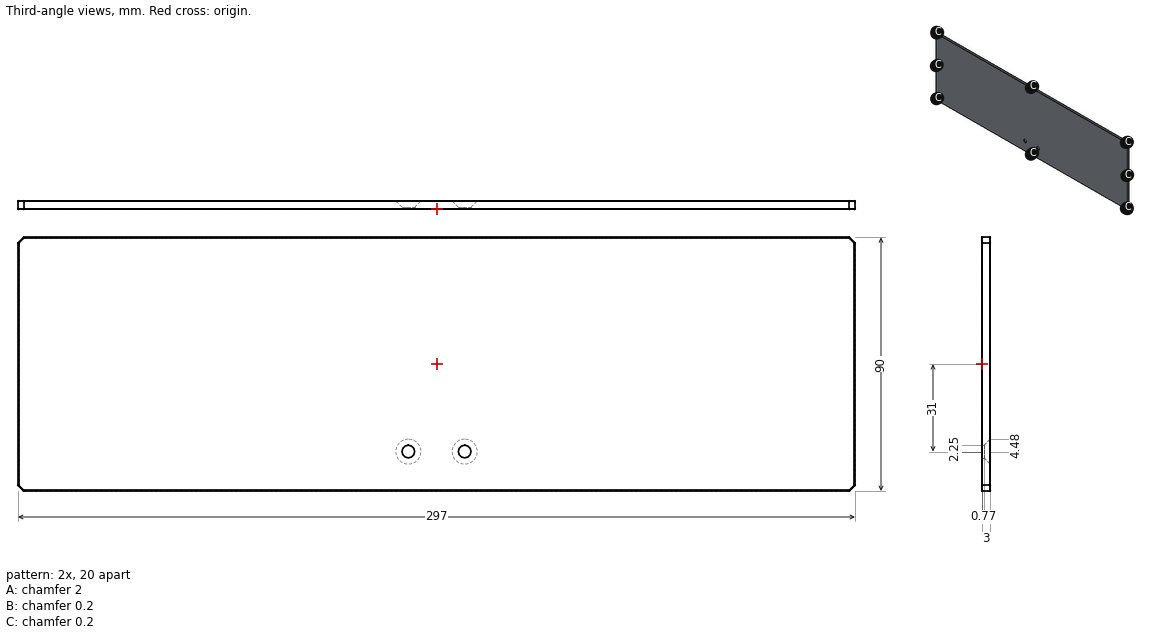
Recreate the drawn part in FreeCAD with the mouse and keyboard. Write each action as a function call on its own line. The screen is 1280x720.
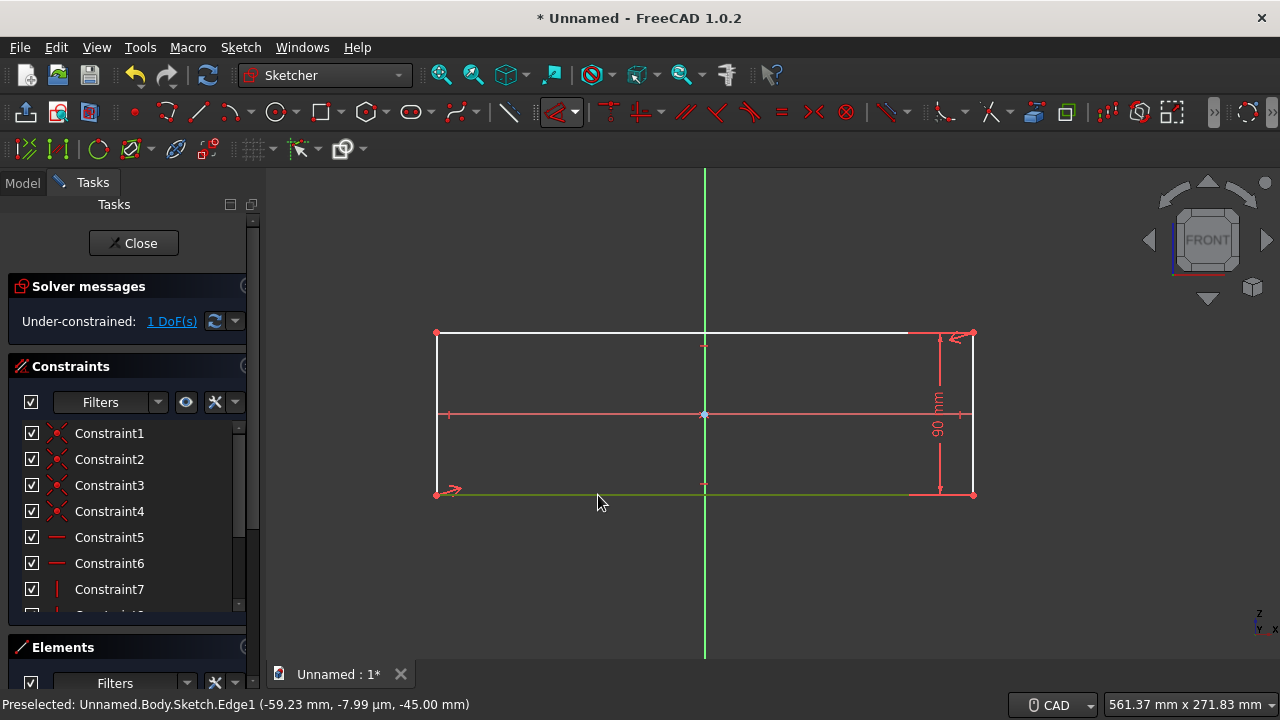
key(l)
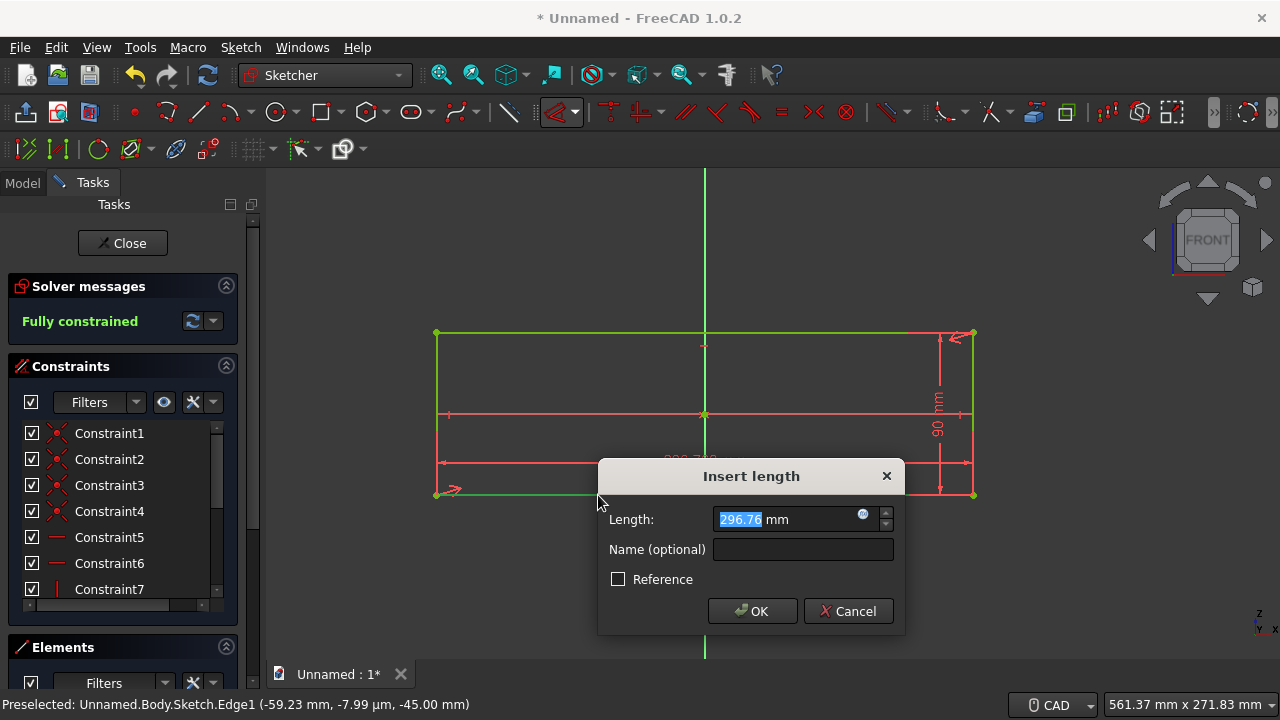
text(297)
key(Return)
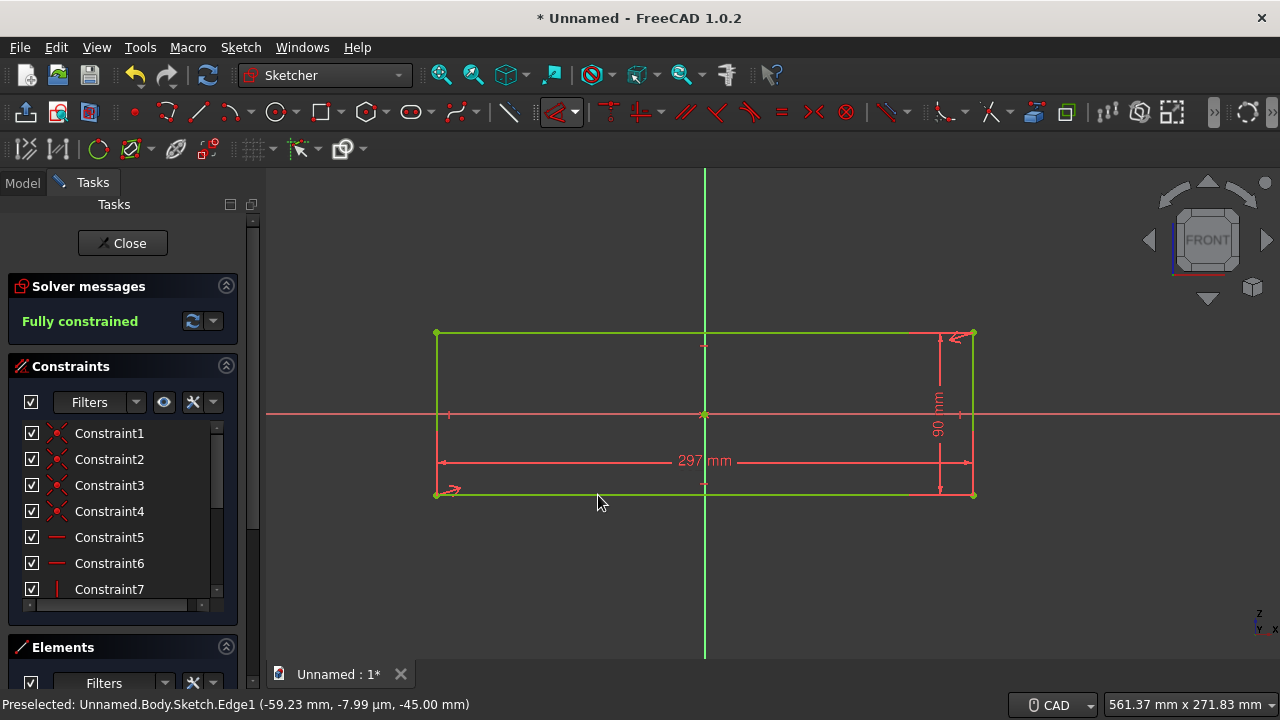
click(123, 243)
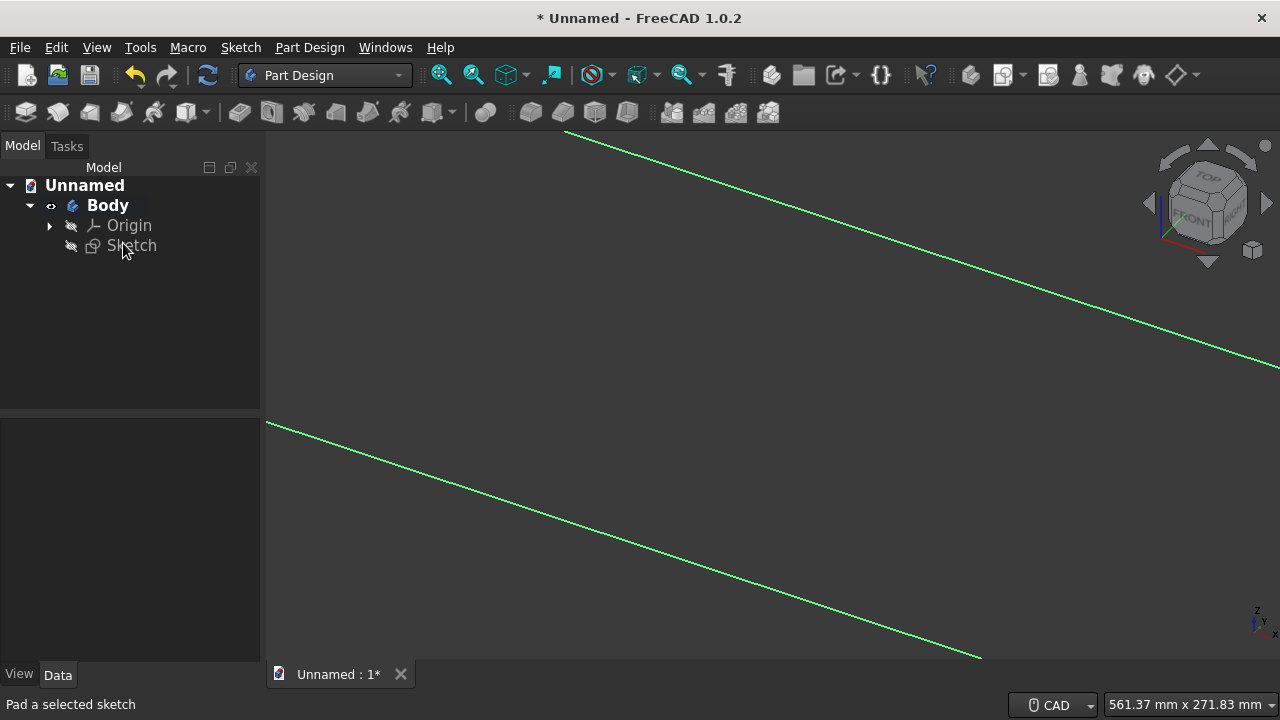
click(26, 112)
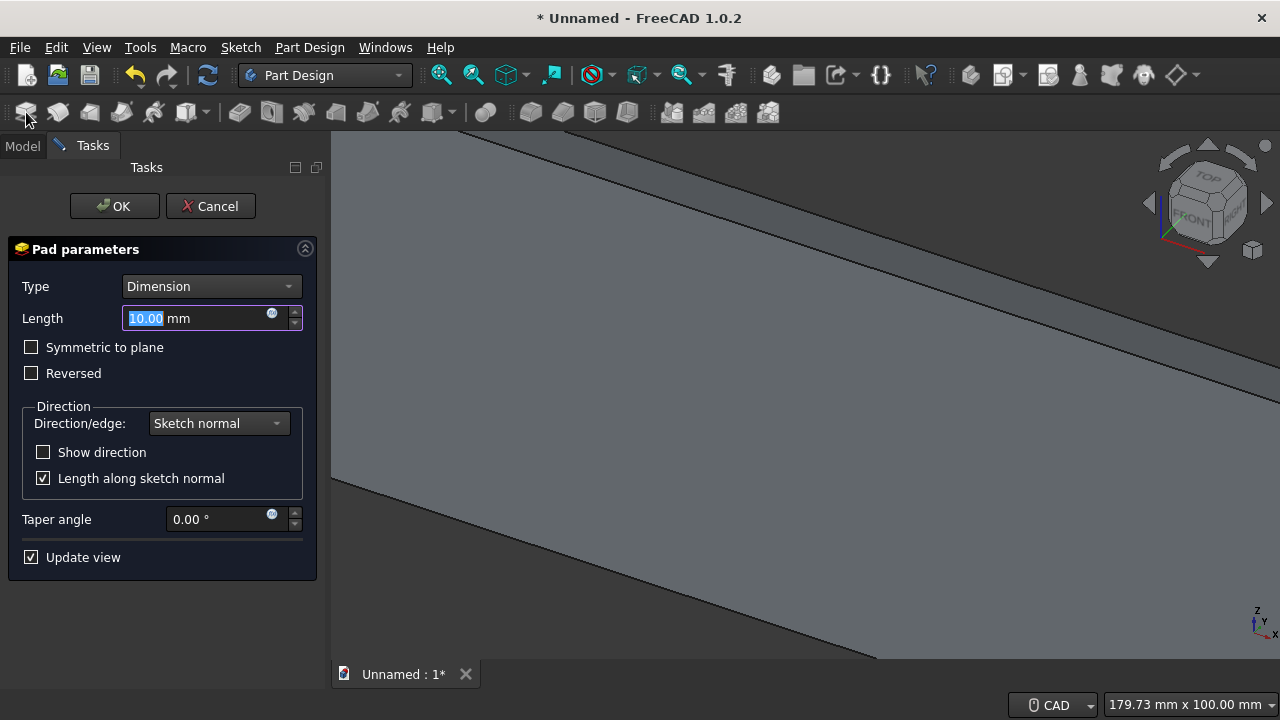
text(3)
key(Tab)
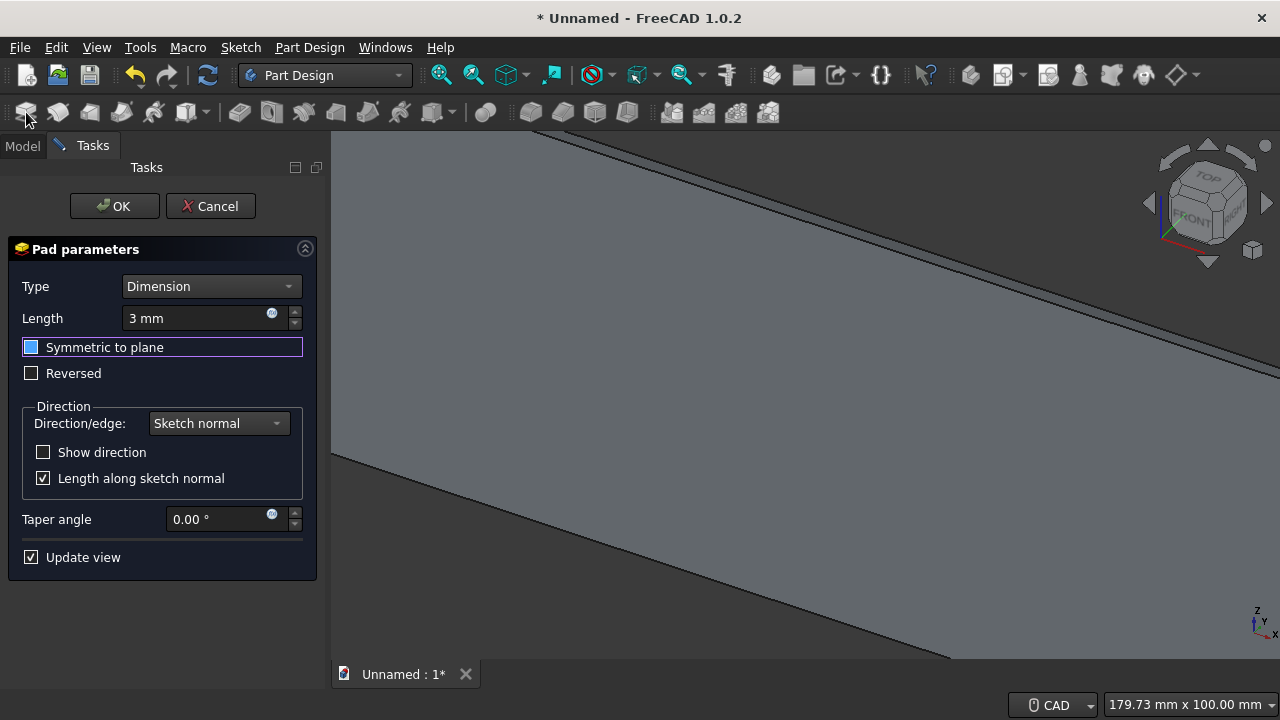
click(30, 373)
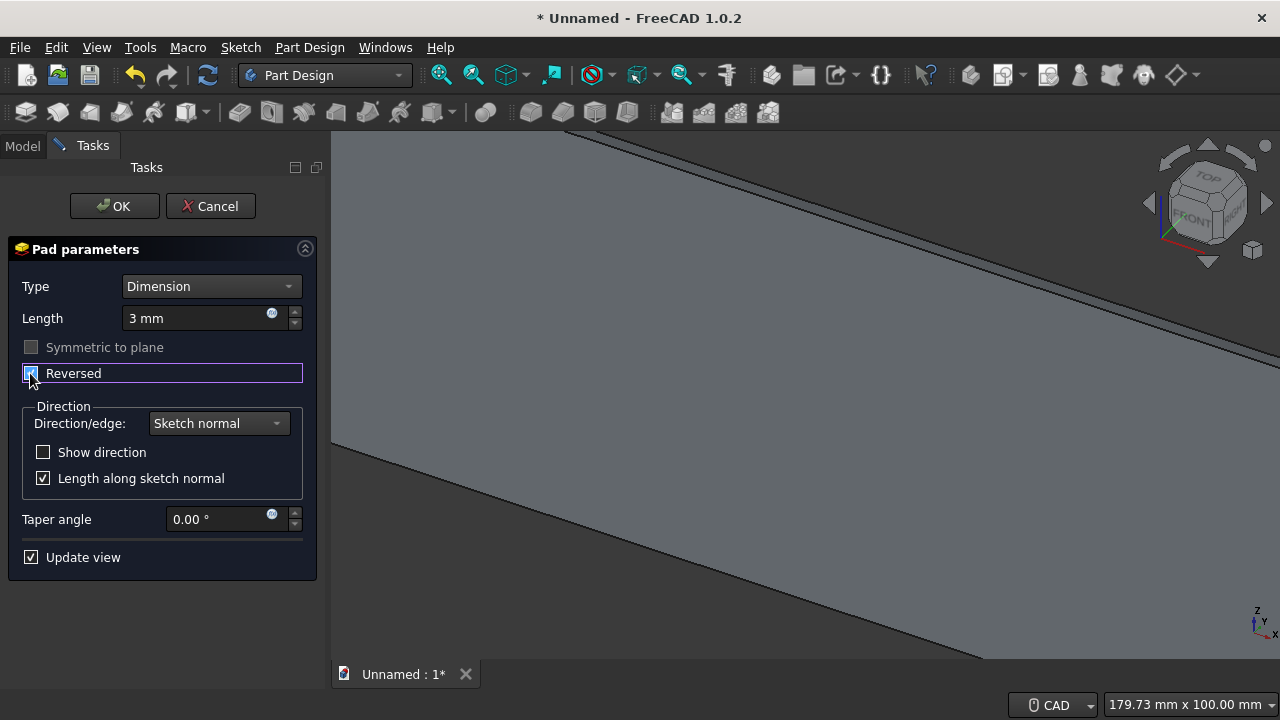
click(115, 206)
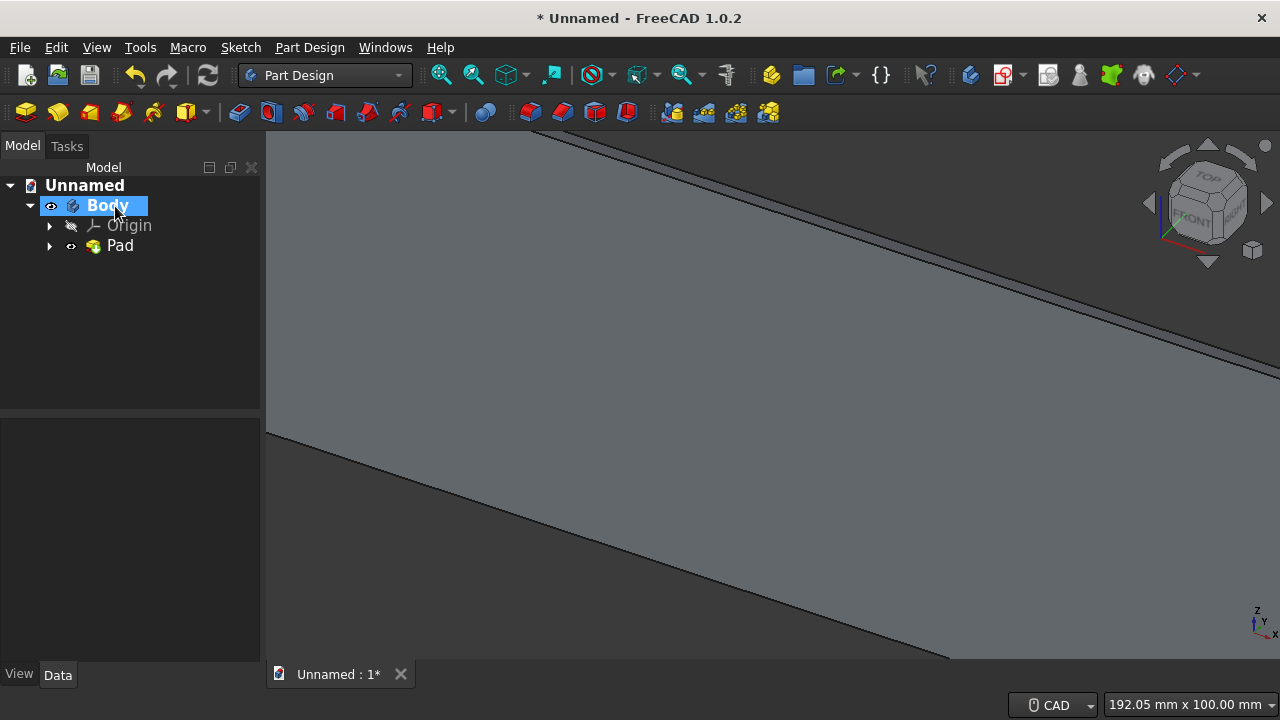
key(v)
key(f)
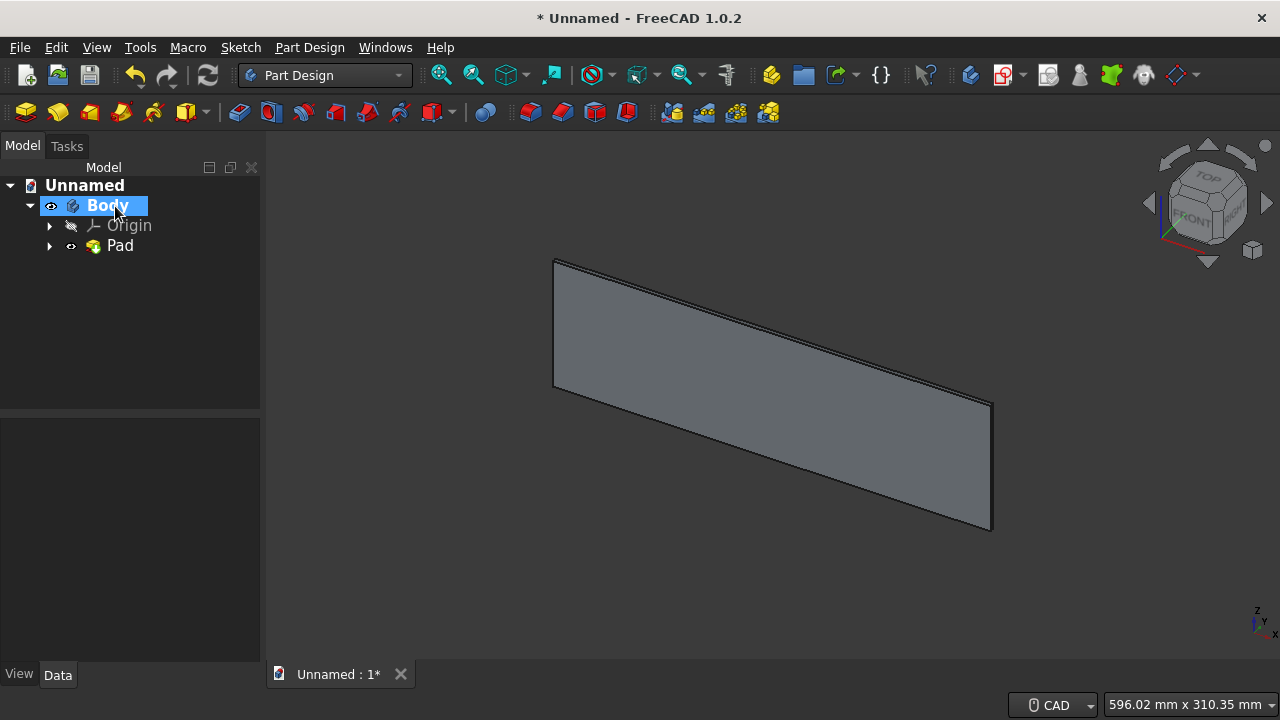
click(50, 226)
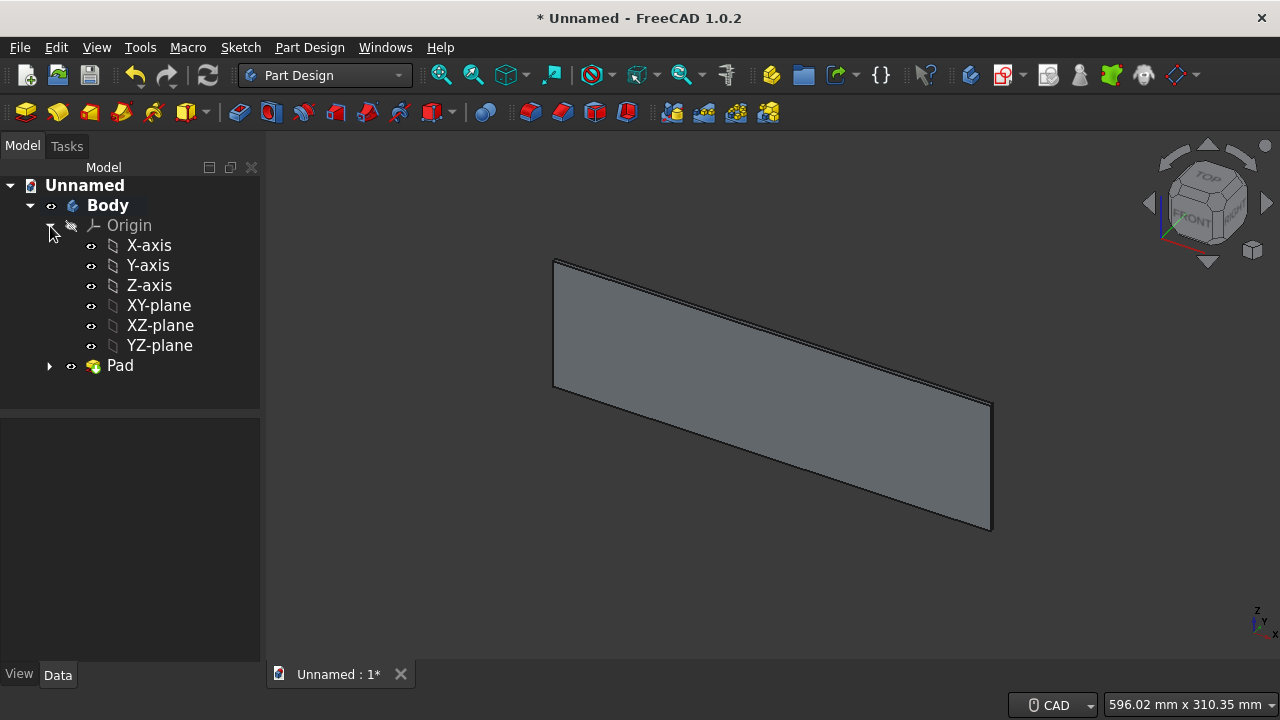
click(136, 346)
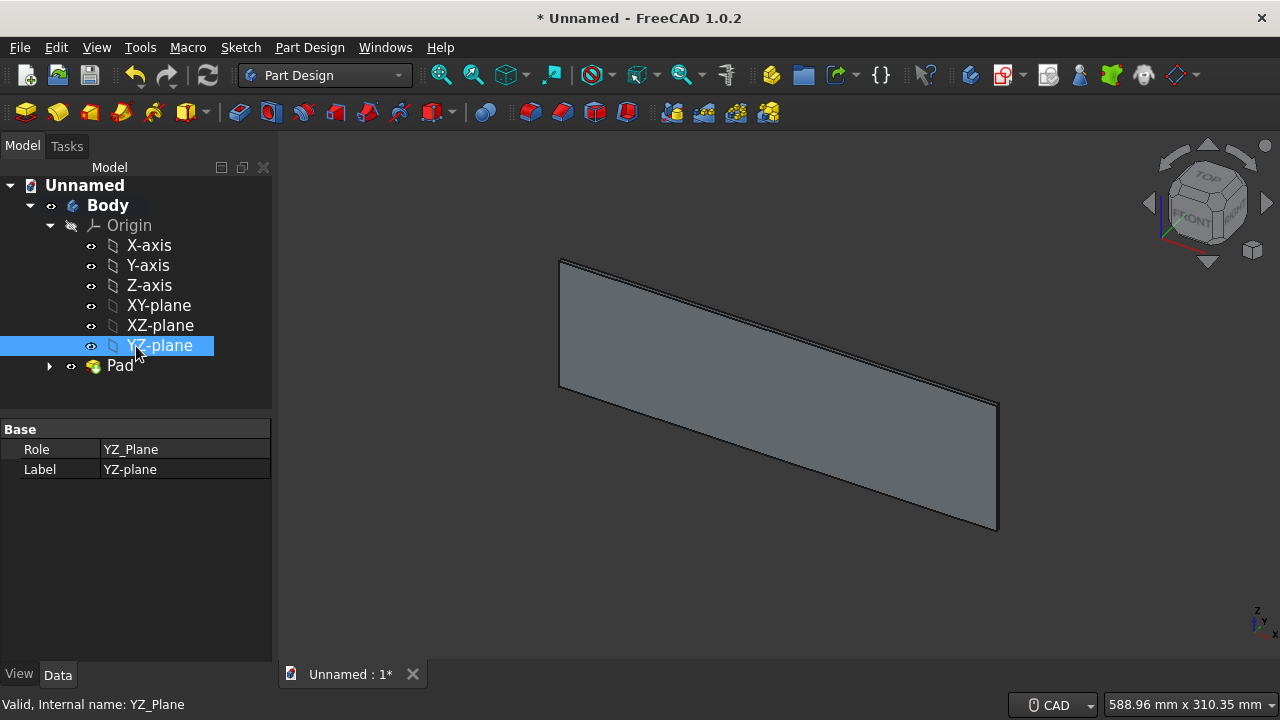
click(1176, 76)